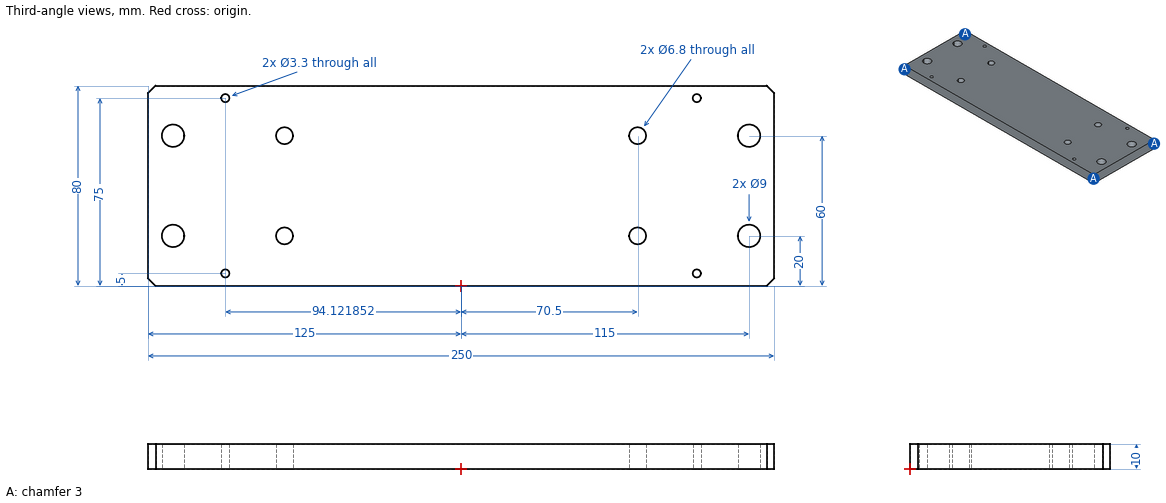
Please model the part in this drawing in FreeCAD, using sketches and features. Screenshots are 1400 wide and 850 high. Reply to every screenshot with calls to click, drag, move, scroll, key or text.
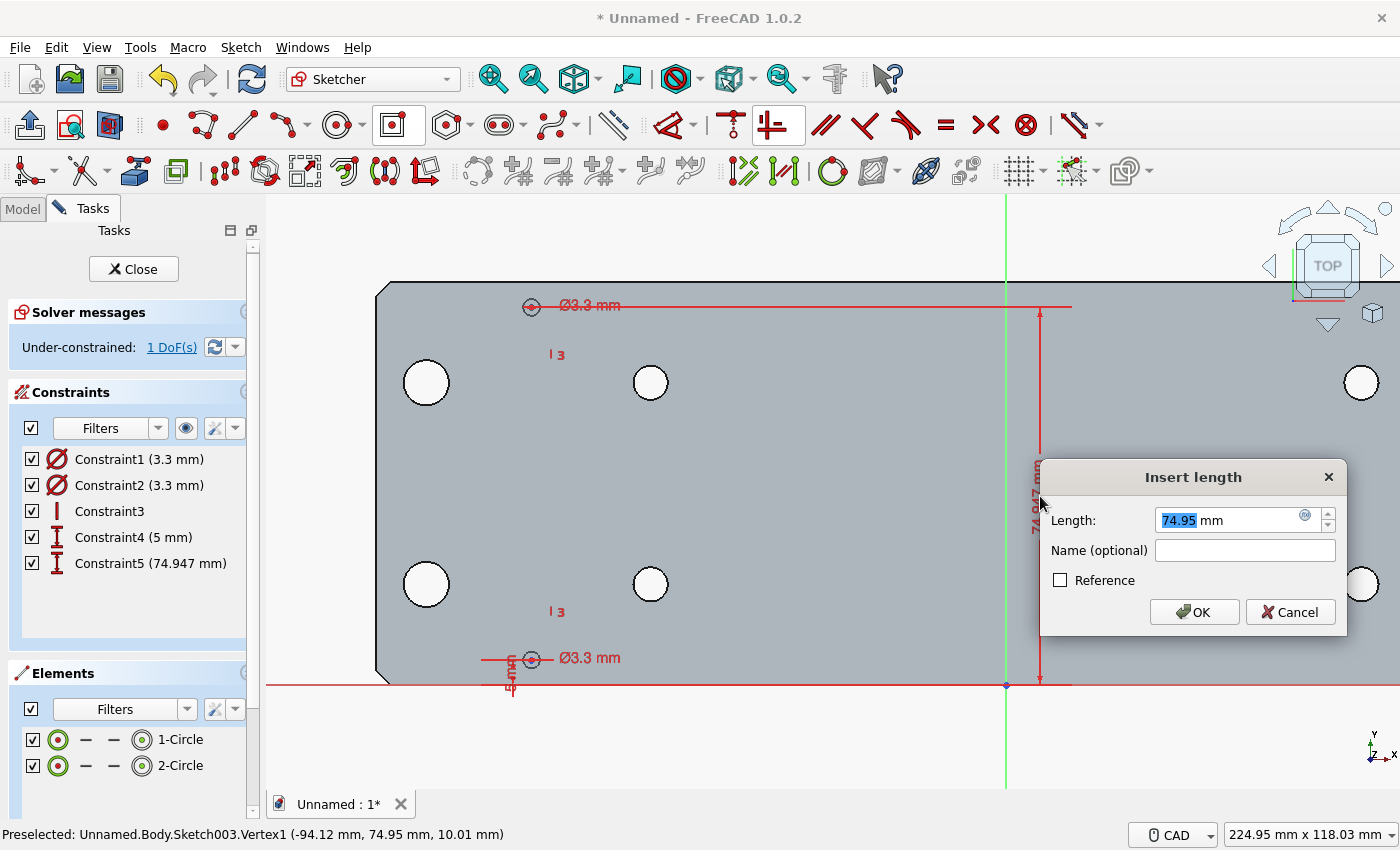
text(75)
key(Return)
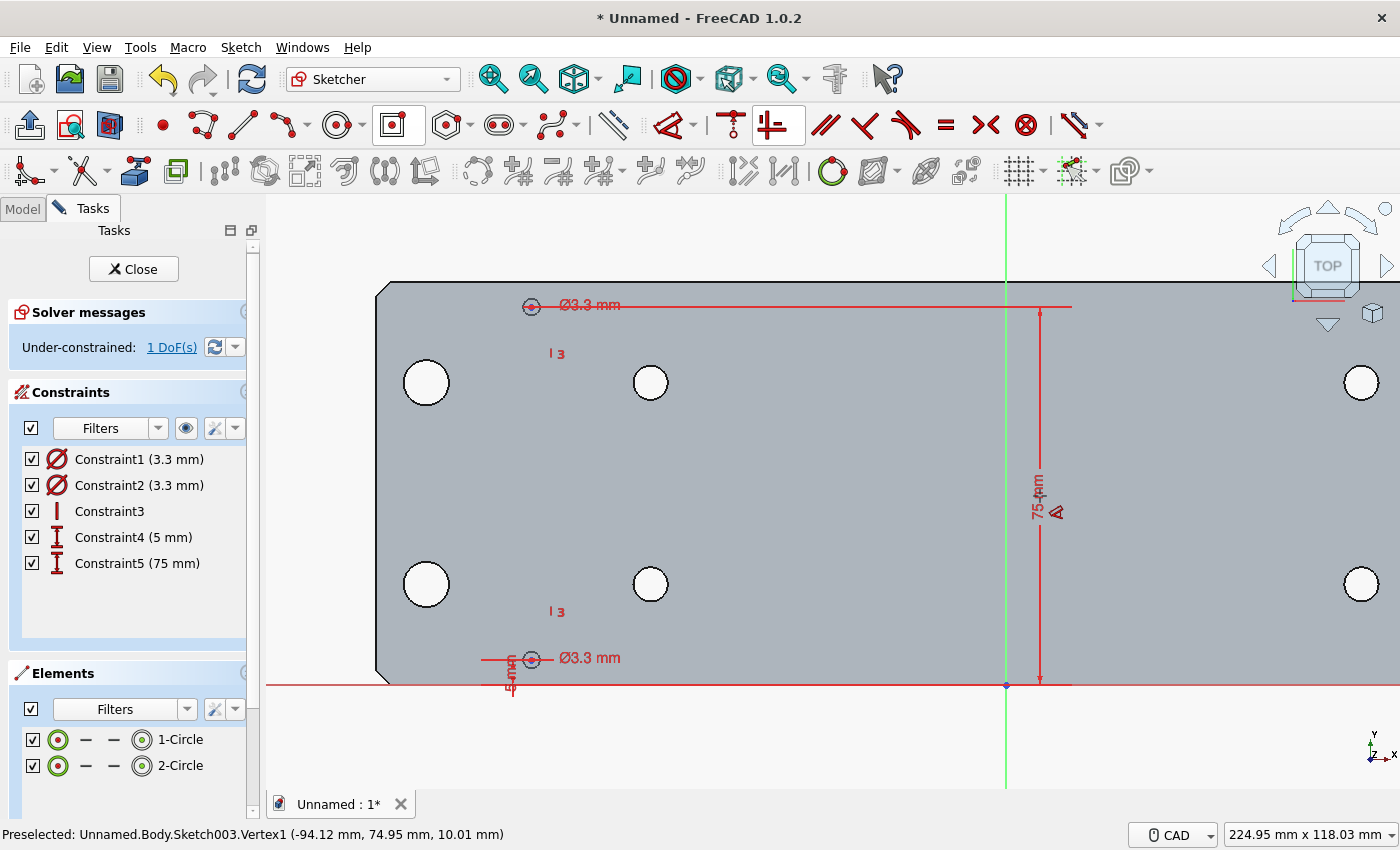
click(532, 307)
click(769, 719)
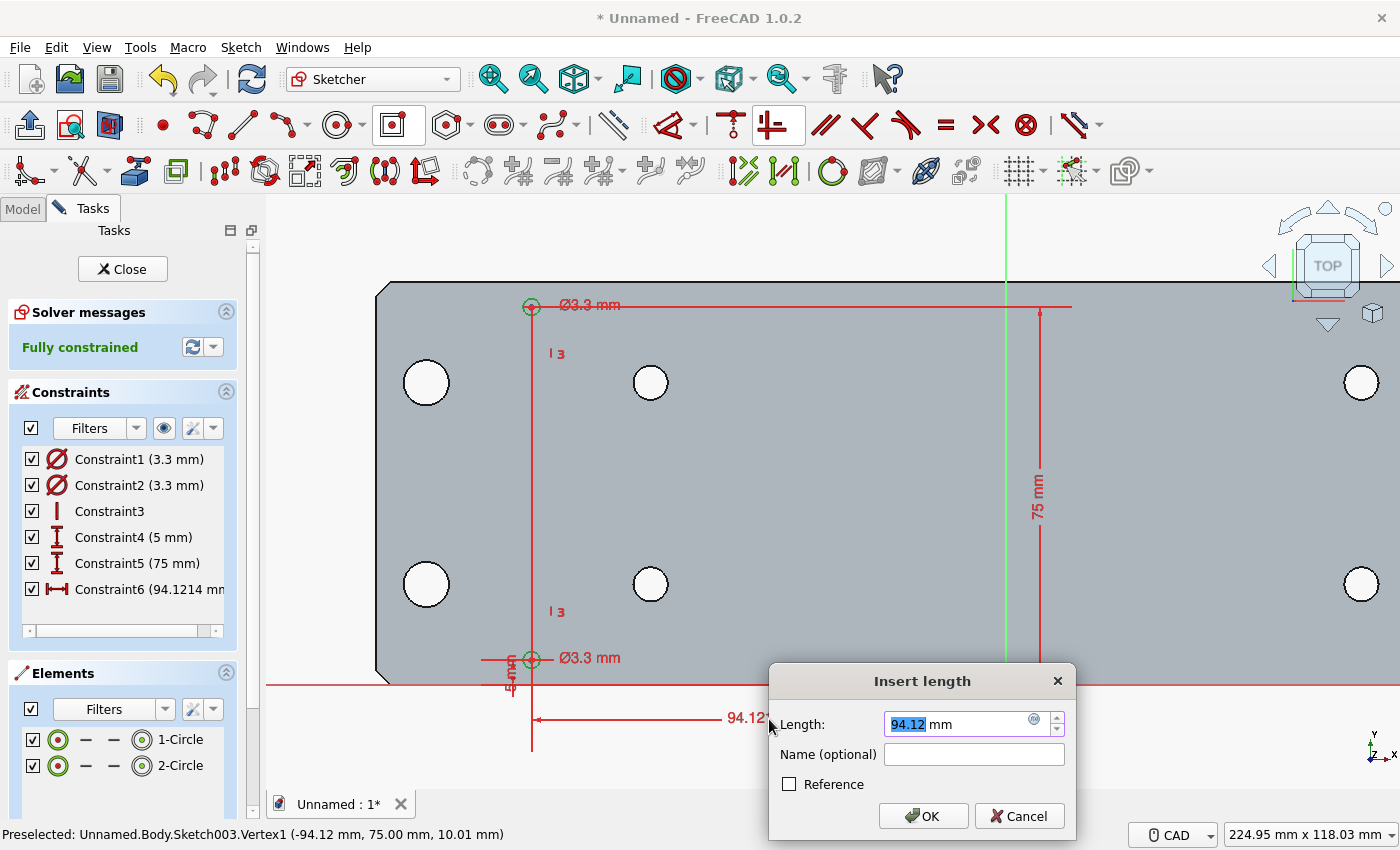
text(94.121852)
key(Return)
key(Escape)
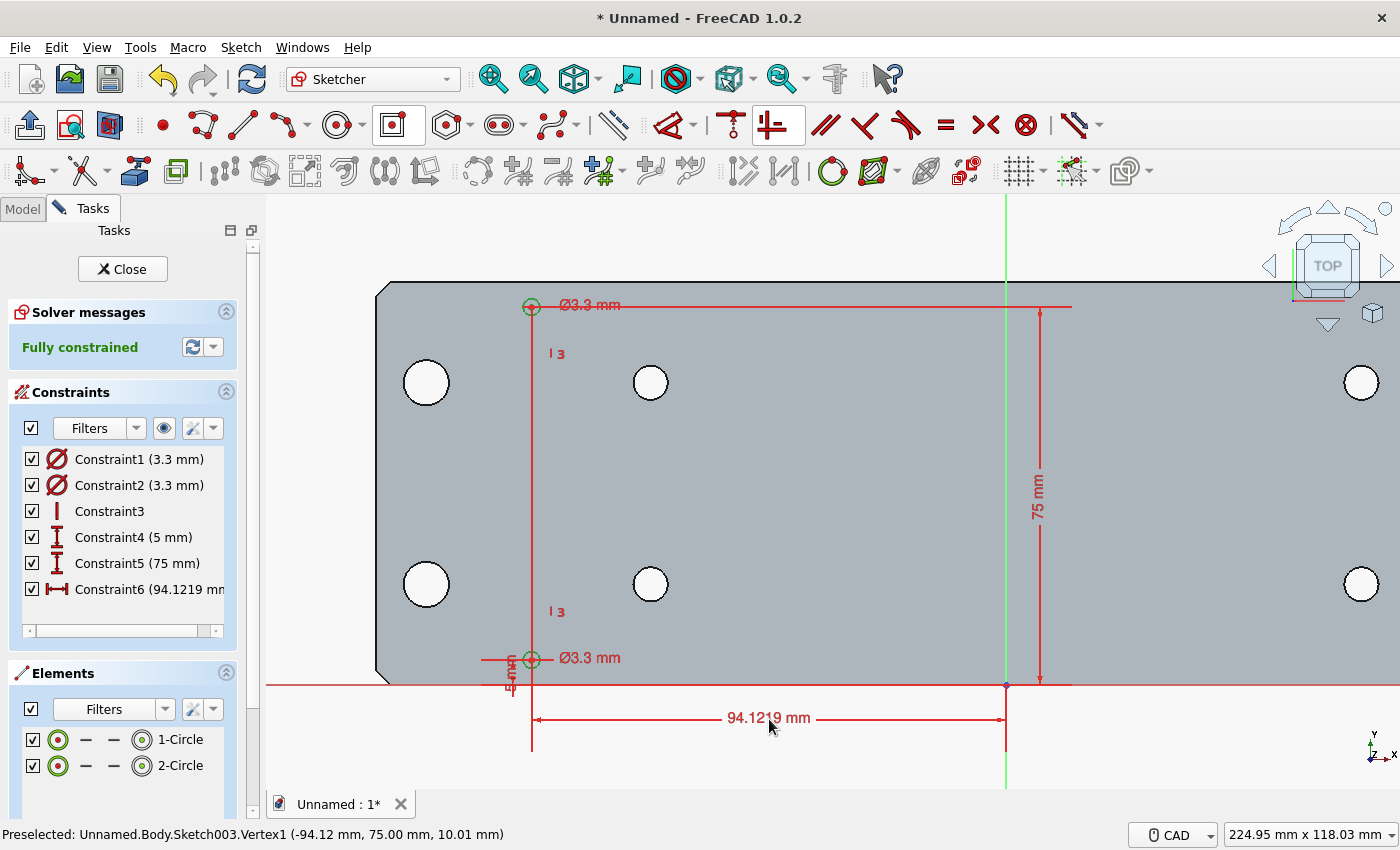
click(123, 269)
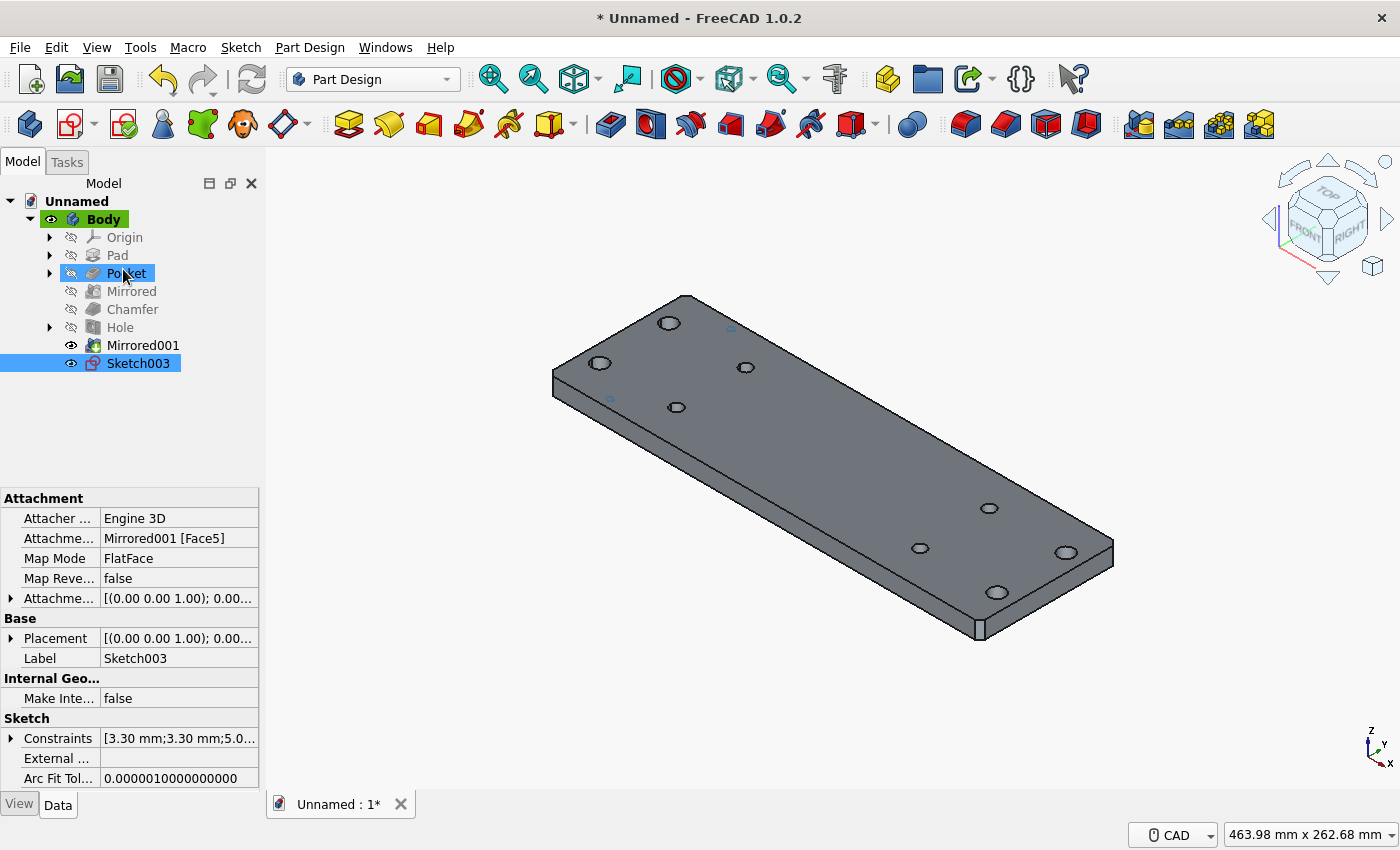
click(652, 124)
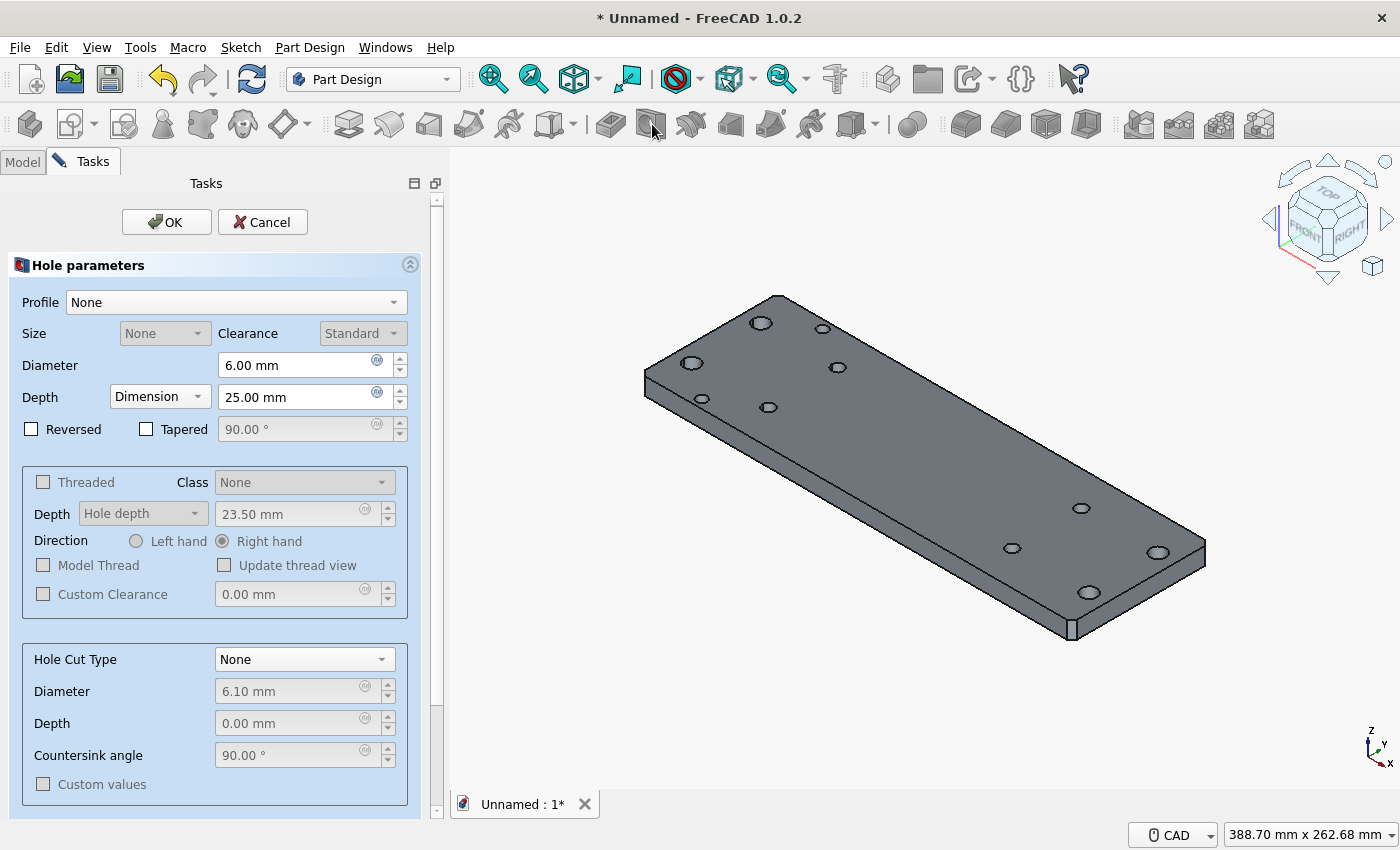
triple_click(305, 365)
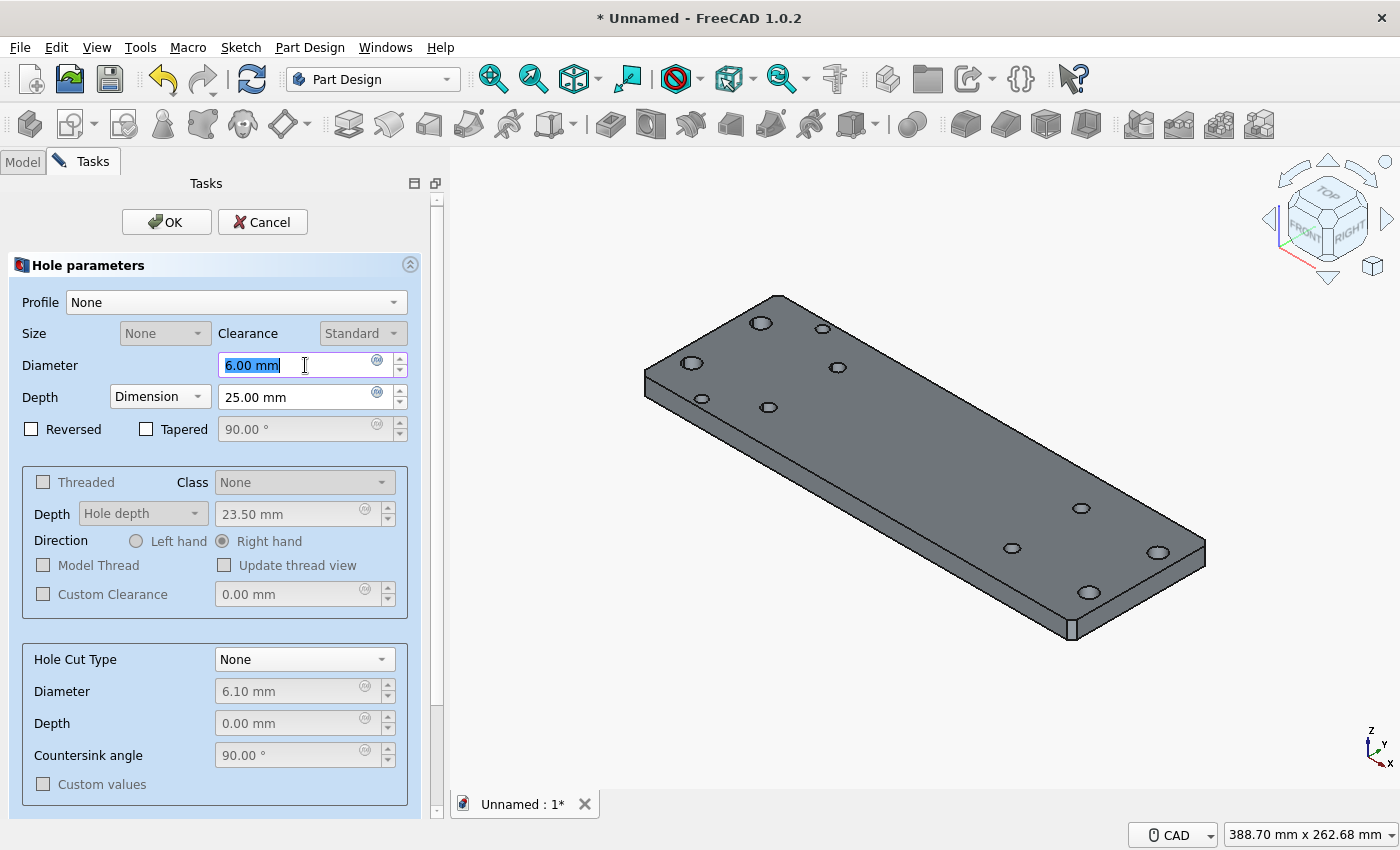
text(3.3)
key(Tab)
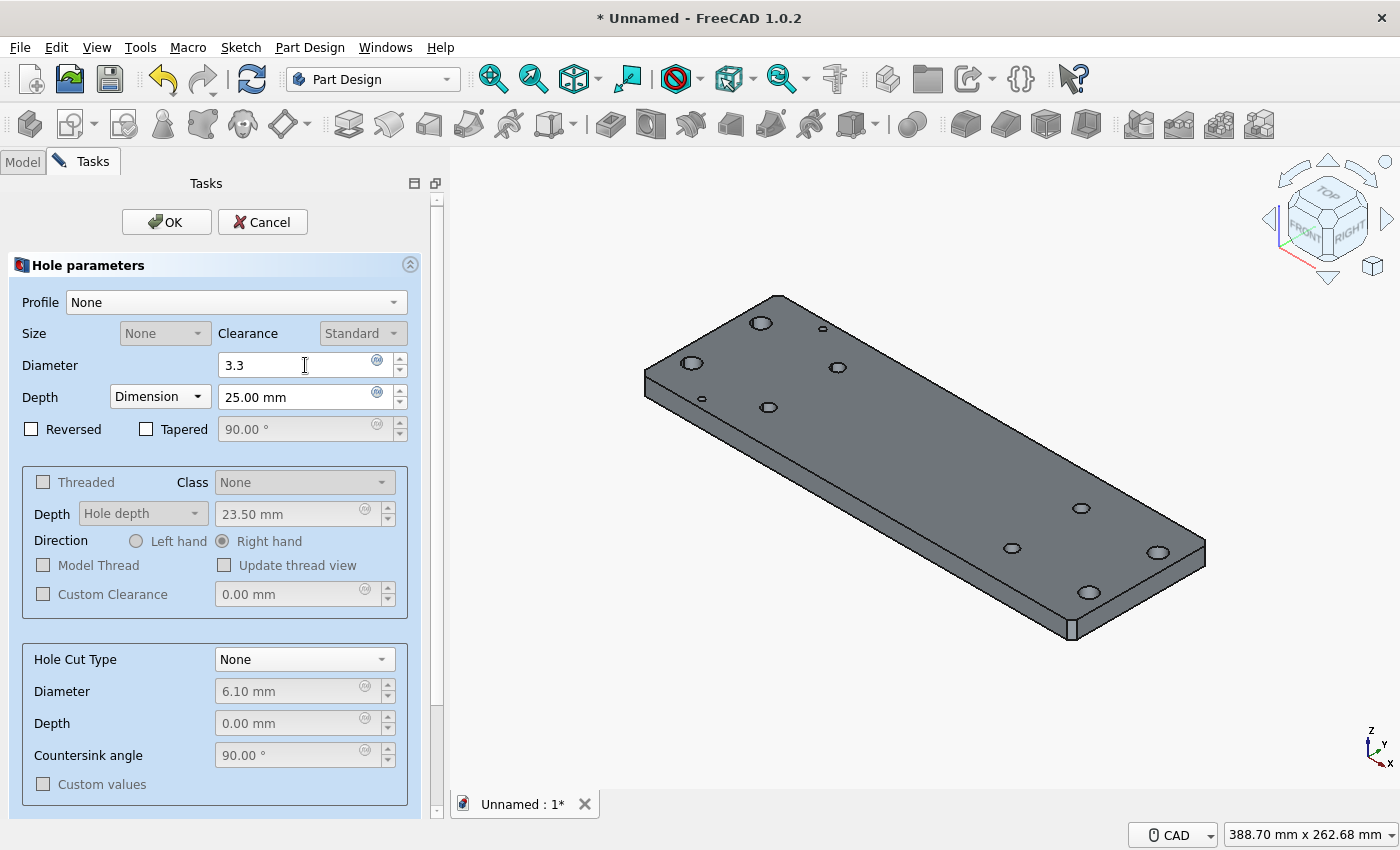
click(161, 396)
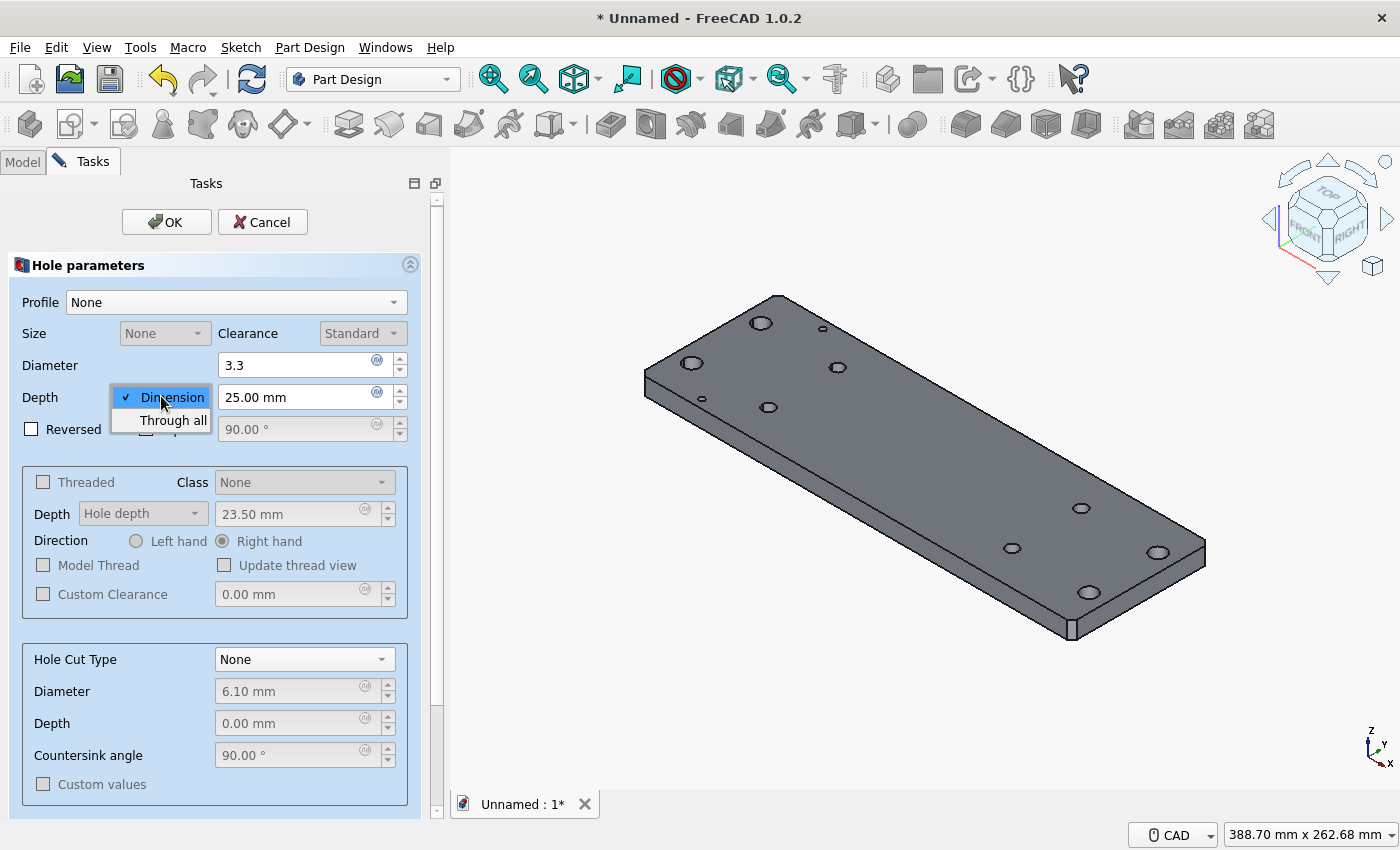
click(160, 420)